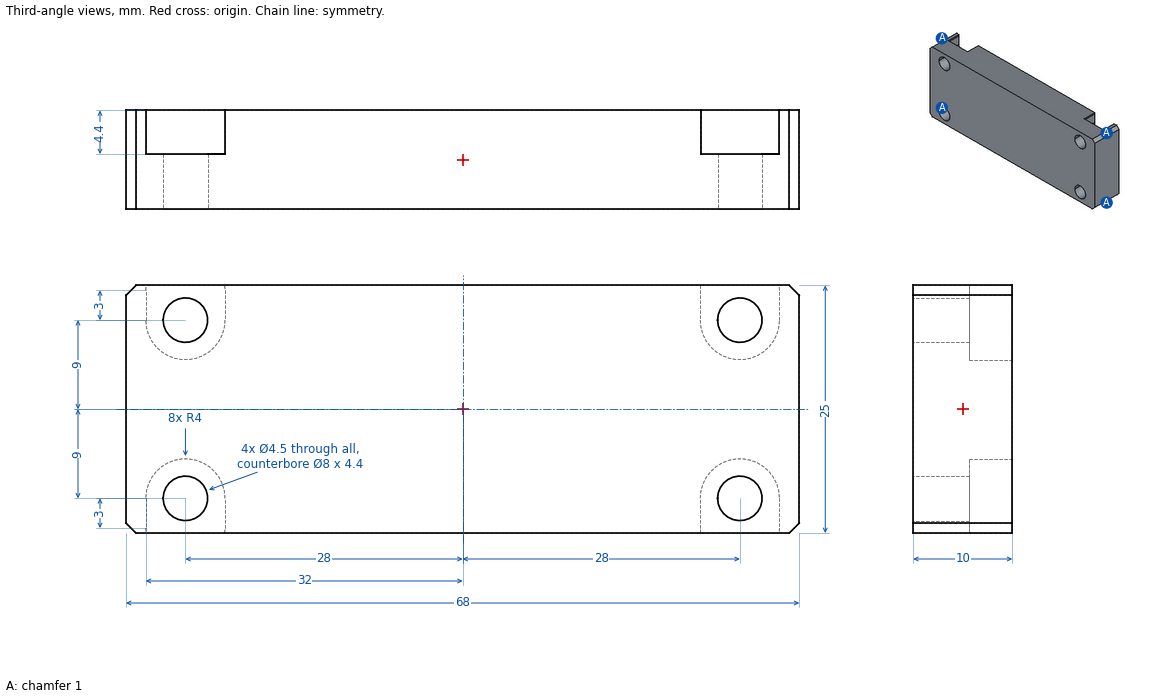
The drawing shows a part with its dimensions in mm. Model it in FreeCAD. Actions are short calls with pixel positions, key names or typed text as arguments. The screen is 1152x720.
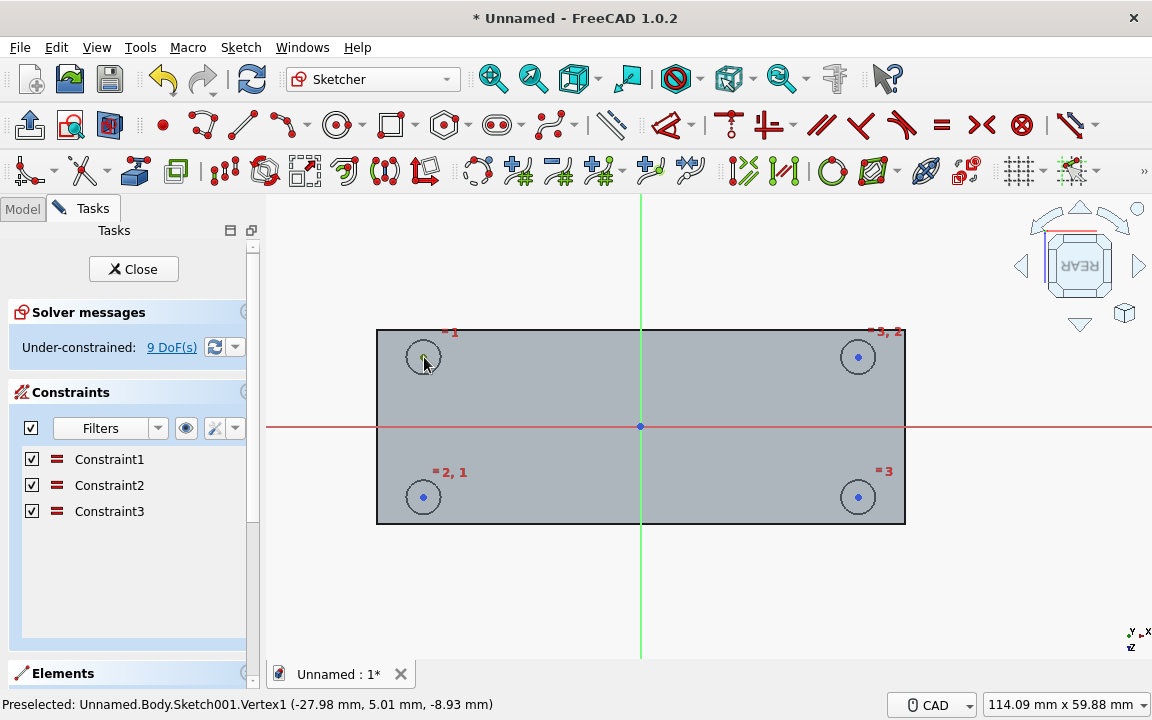
click(424, 497)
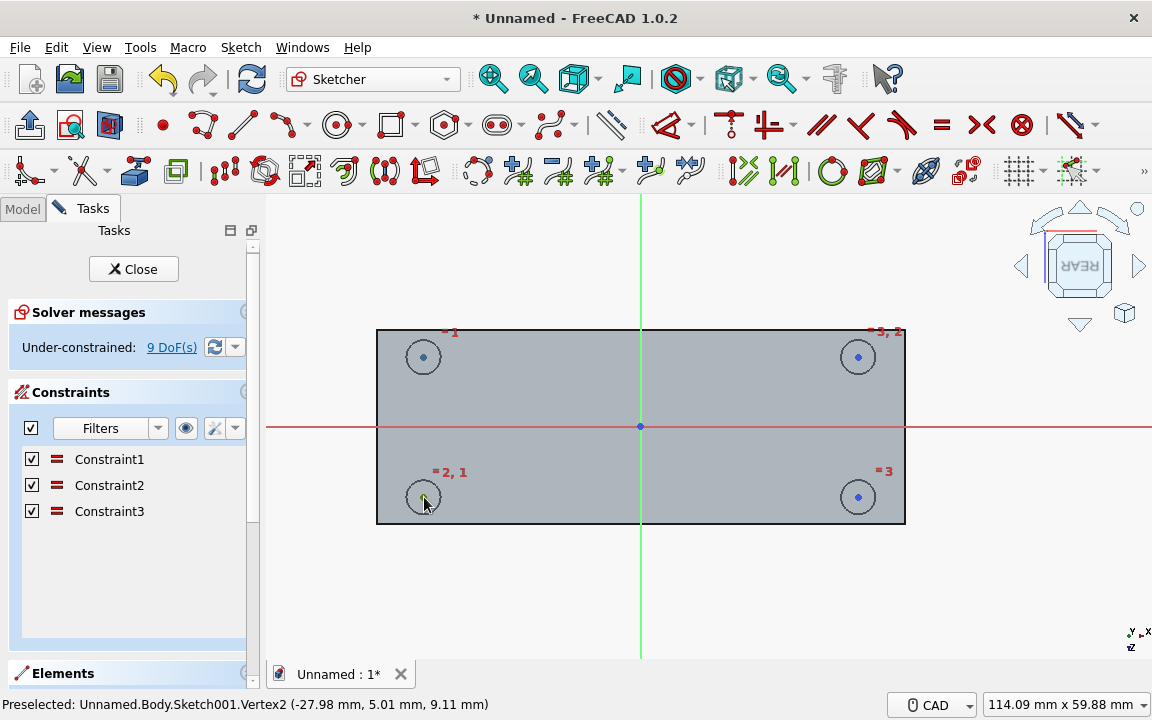
key(v)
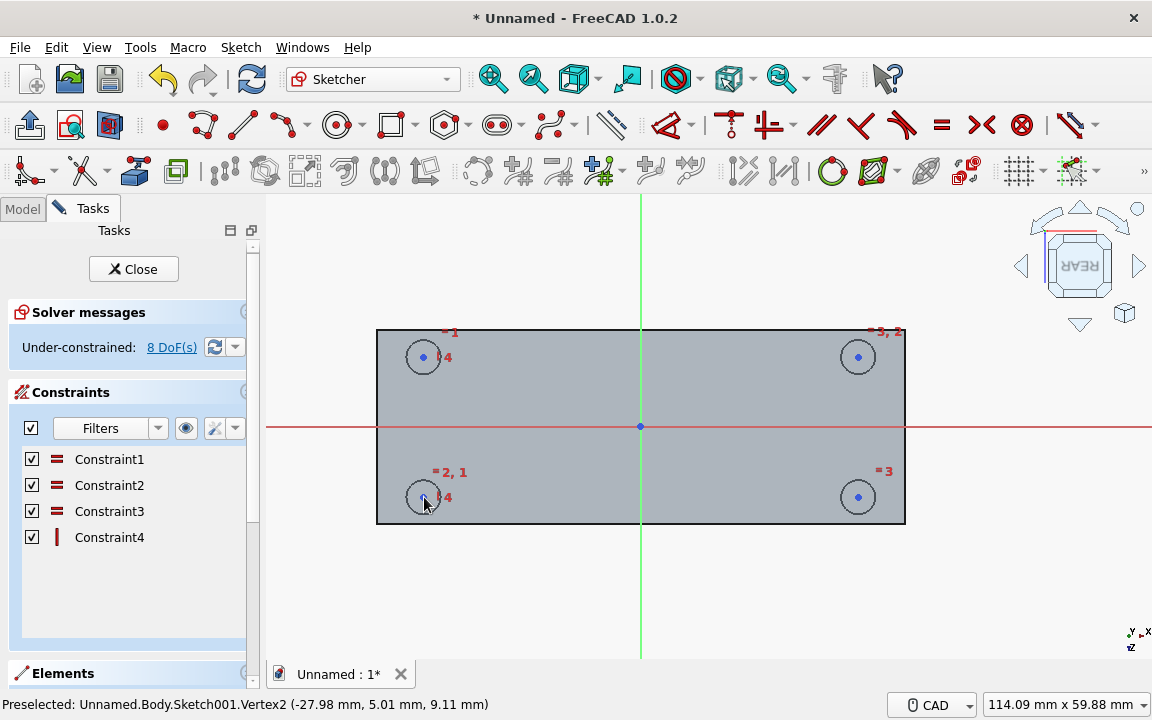
click(424, 357)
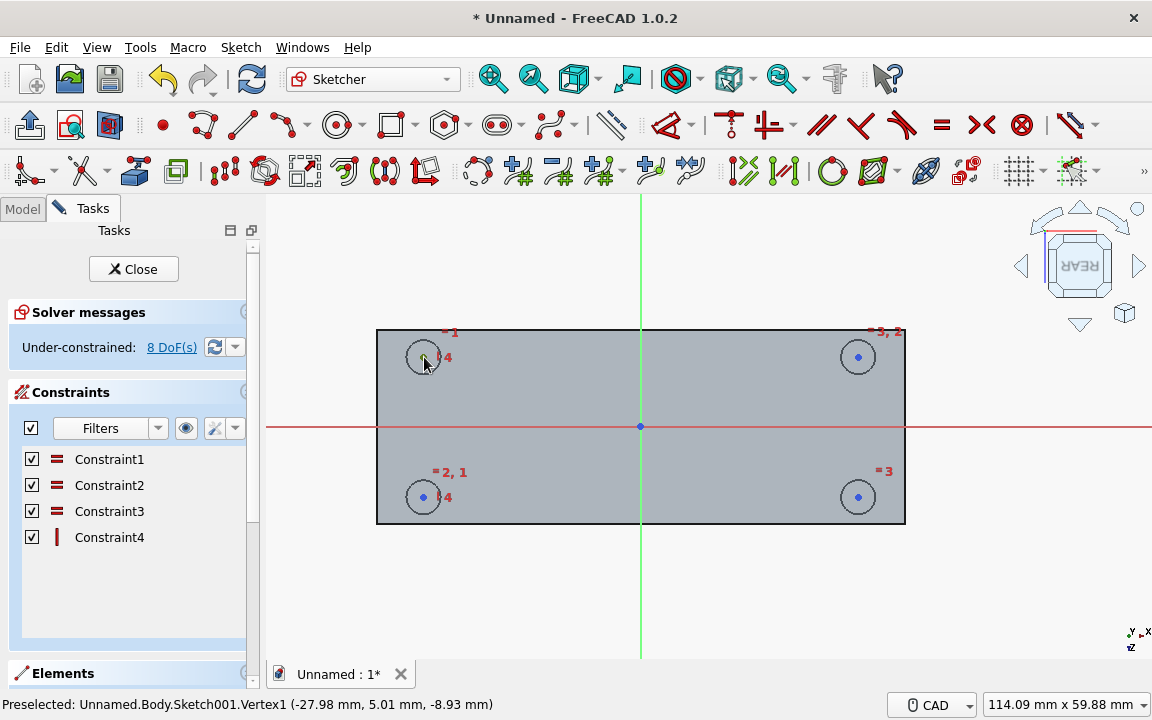
click(858, 357)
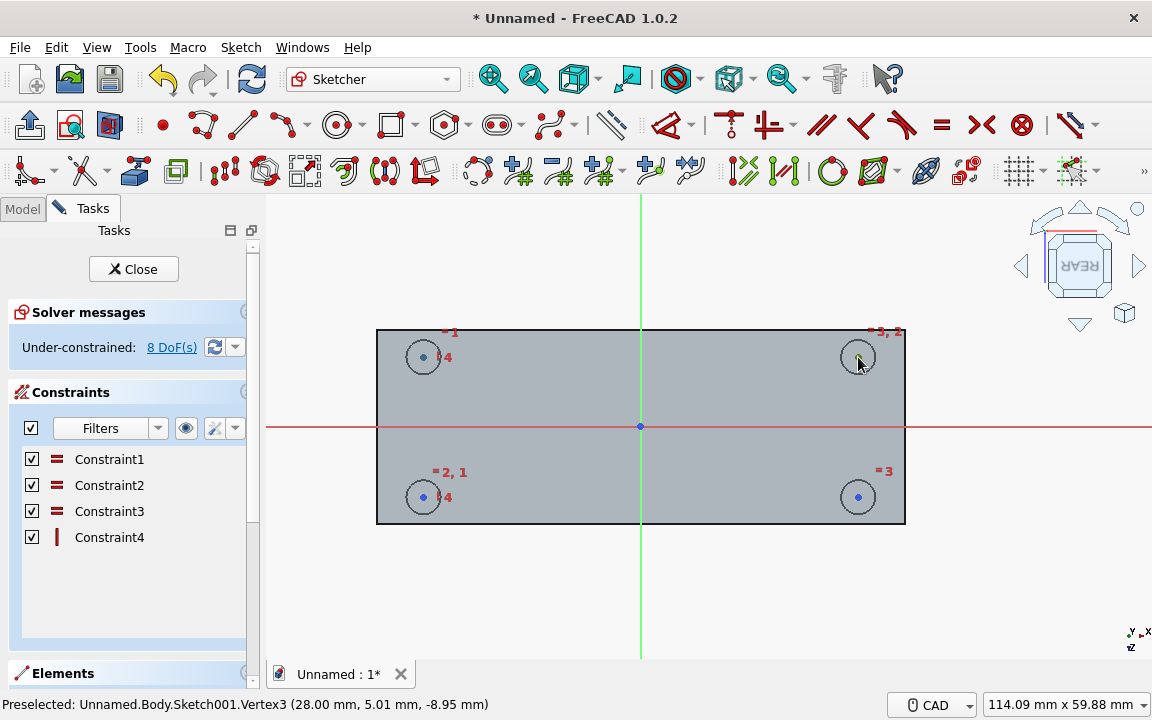
click(796, 126)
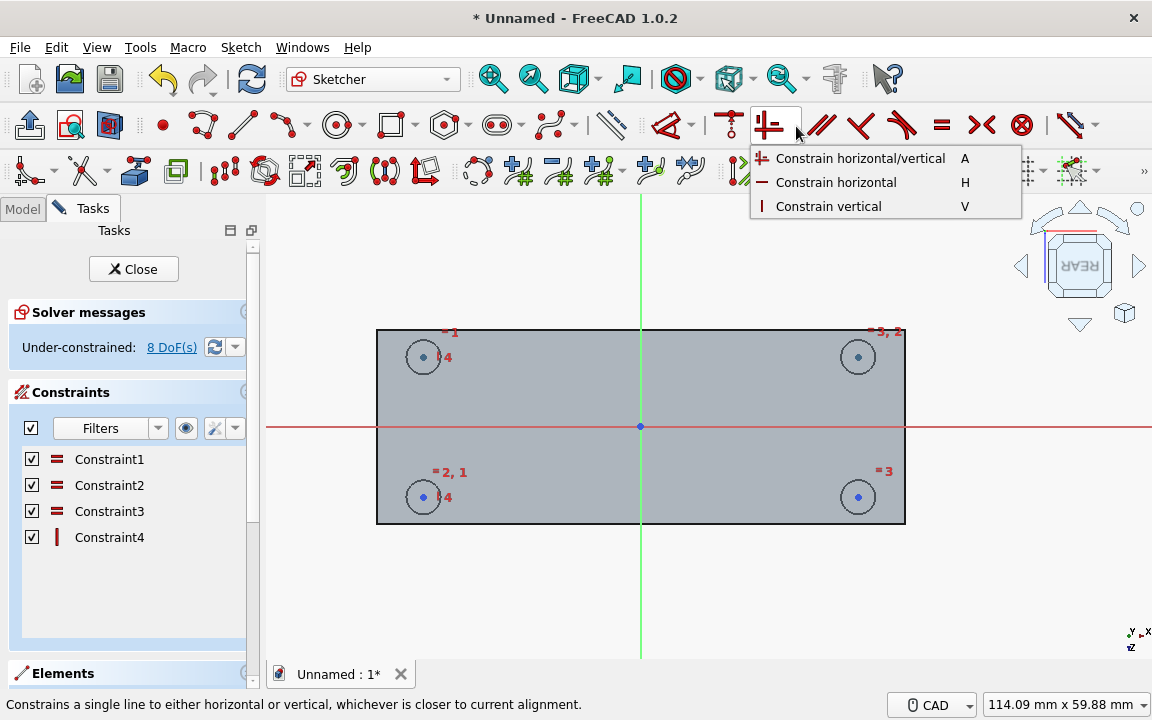
click(886, 182)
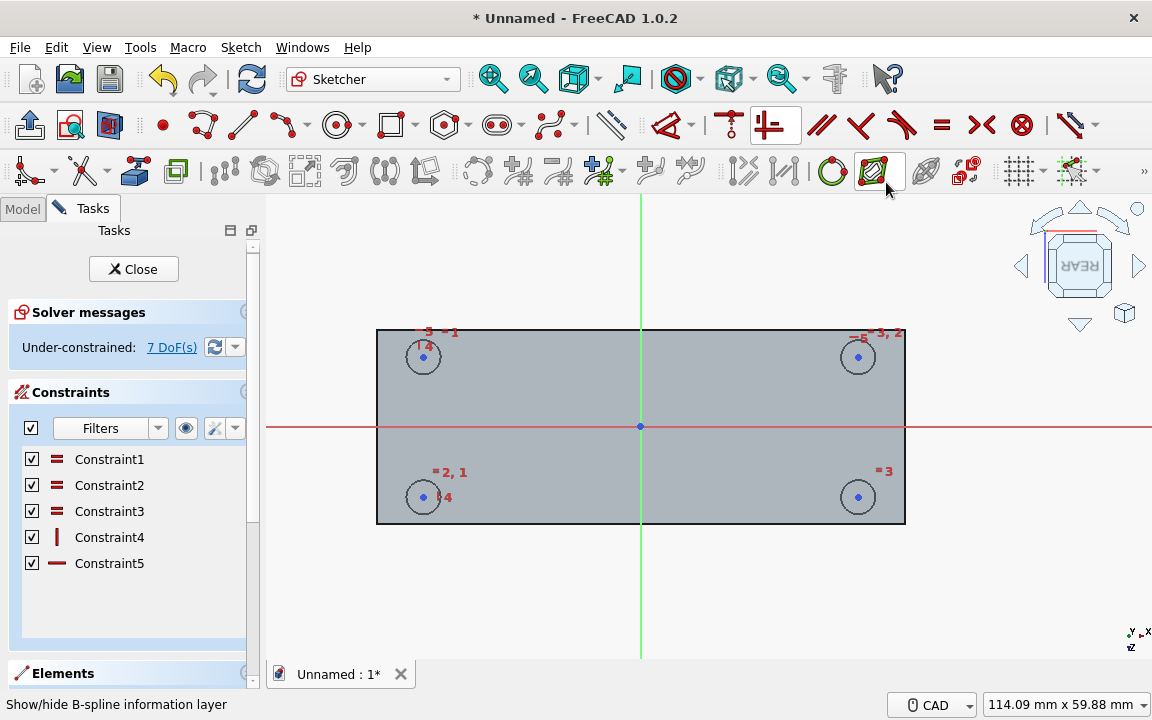
click(858, 357)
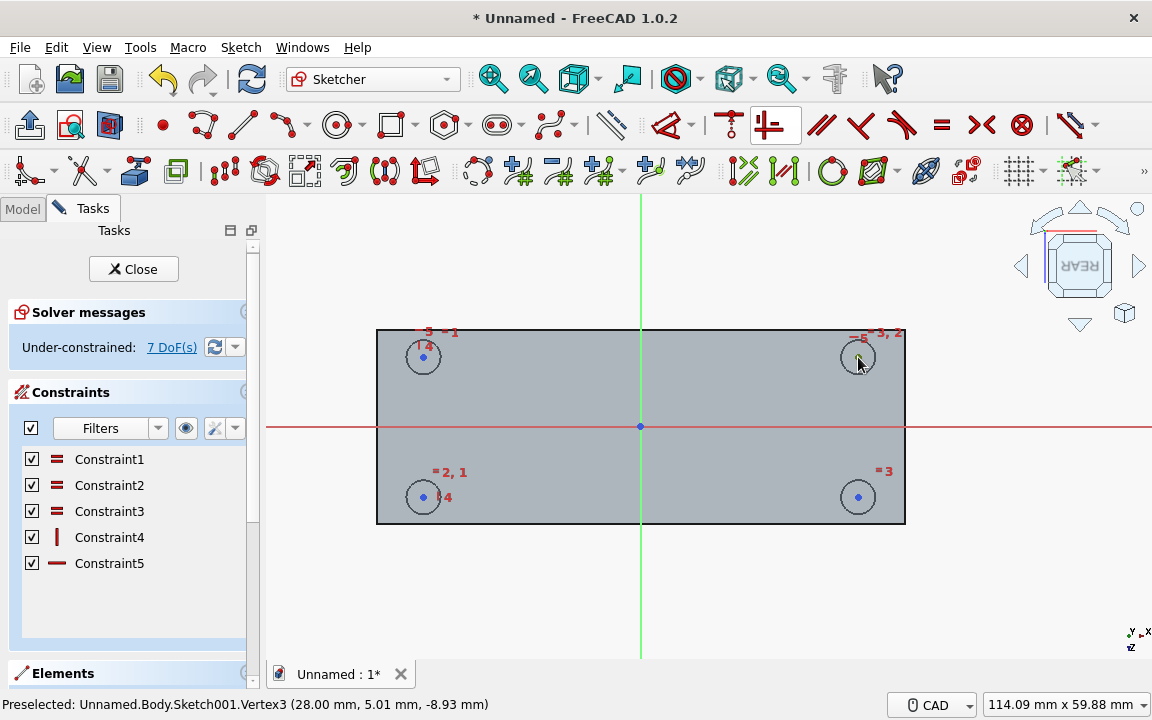
click(858, 497)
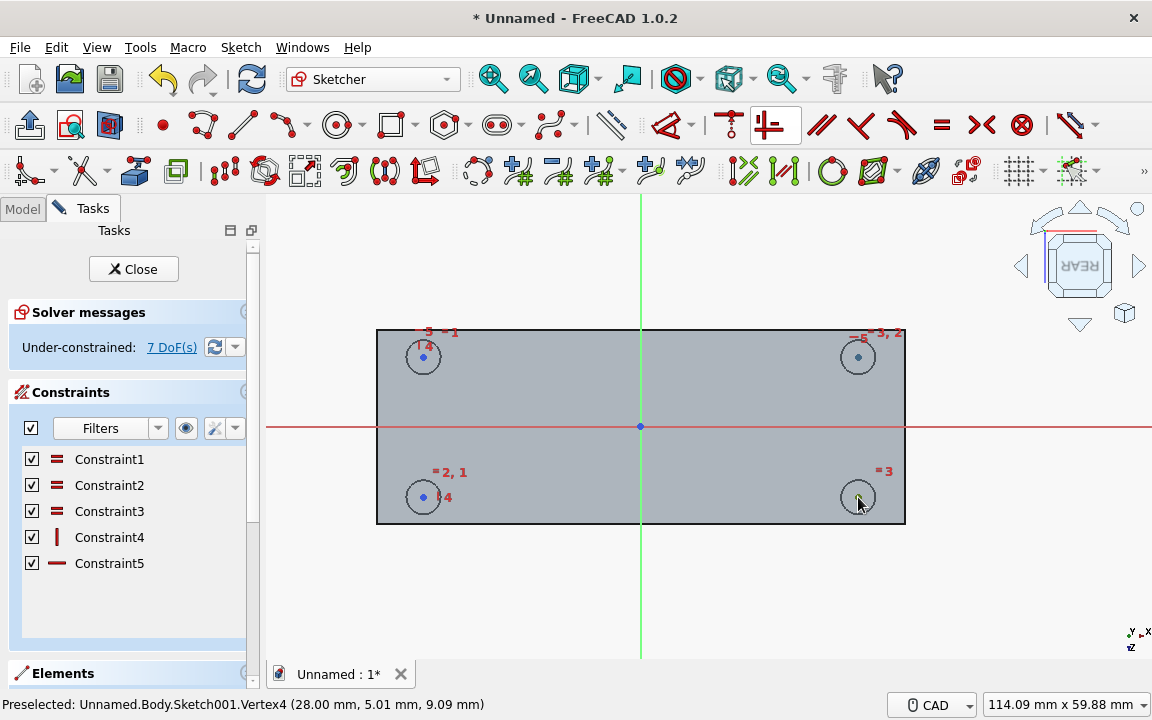
click(796, 126)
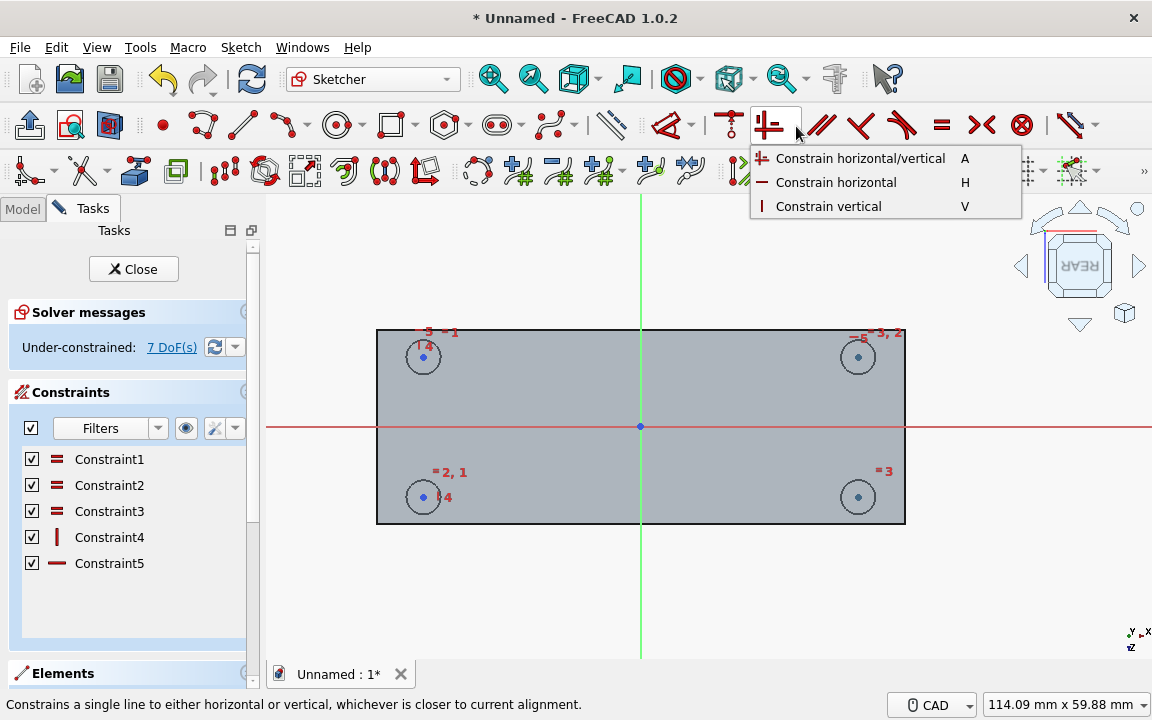
click(886, 206)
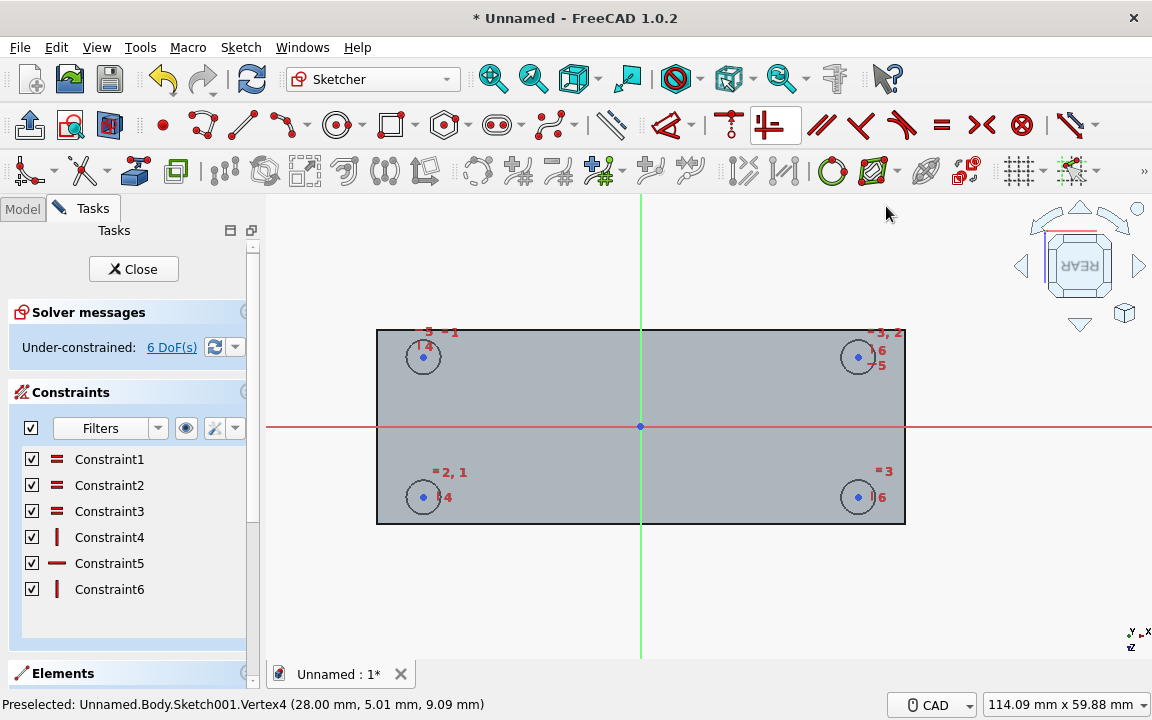
click(424, 497)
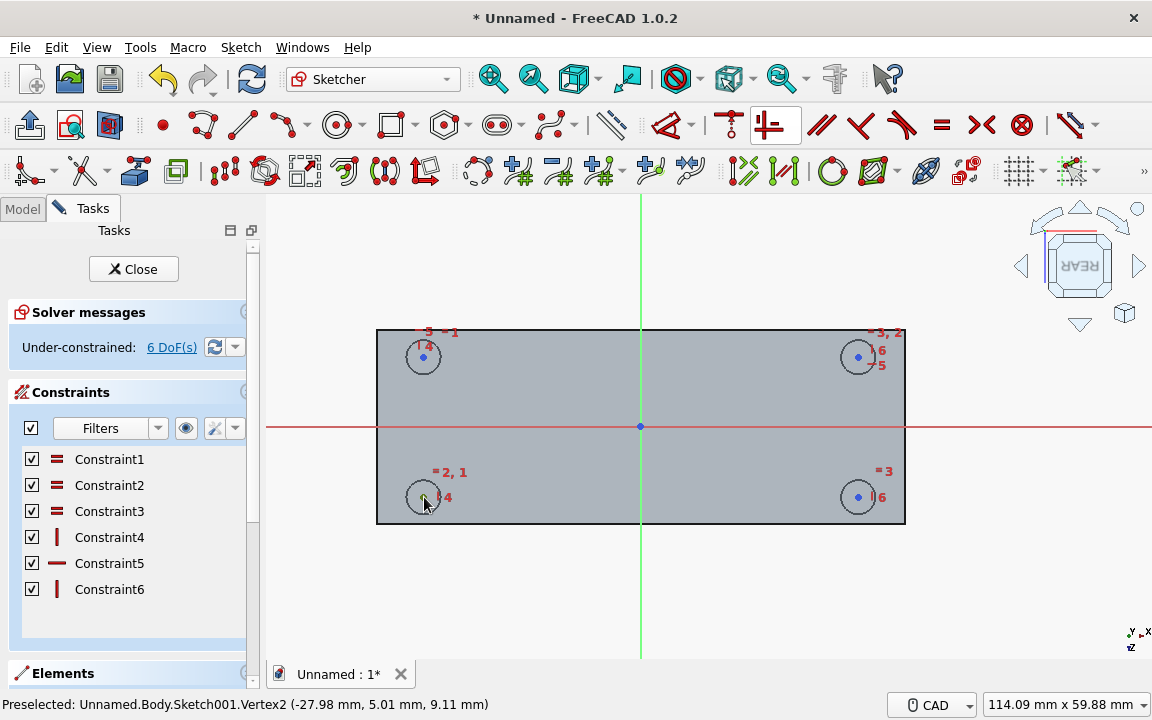
click(858, 497)